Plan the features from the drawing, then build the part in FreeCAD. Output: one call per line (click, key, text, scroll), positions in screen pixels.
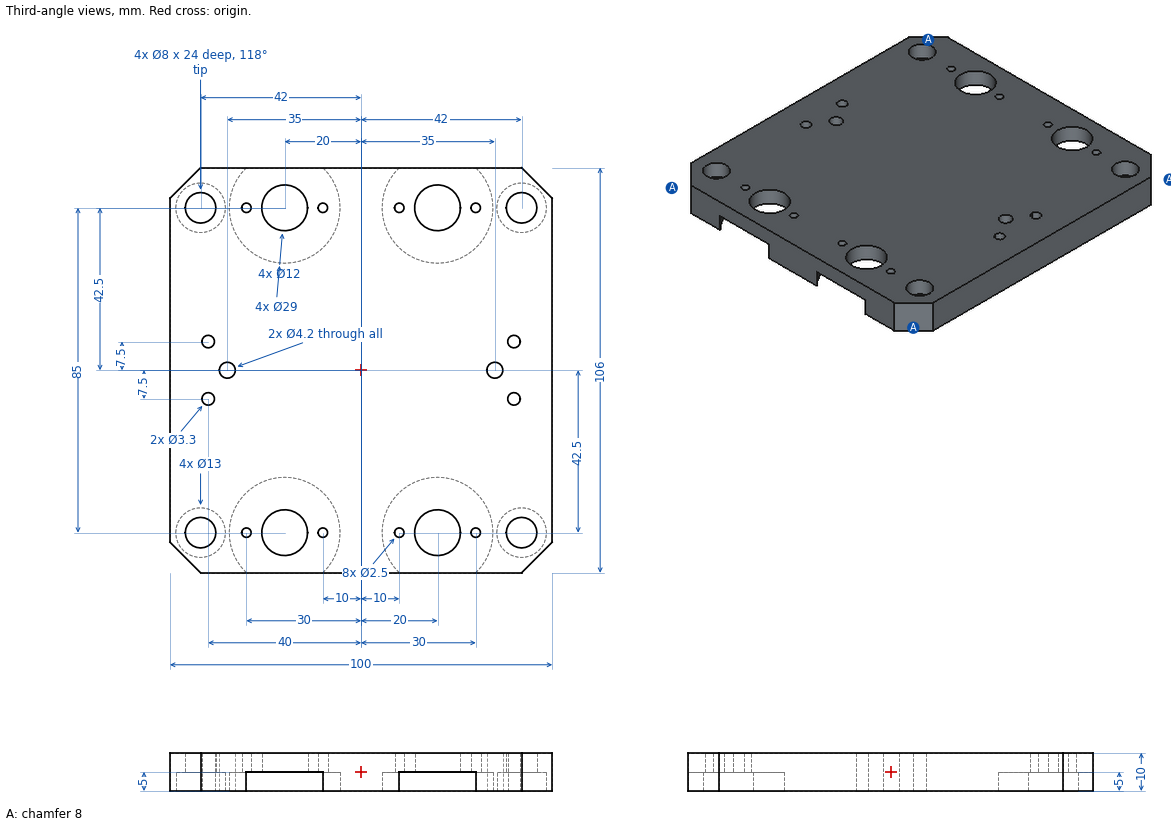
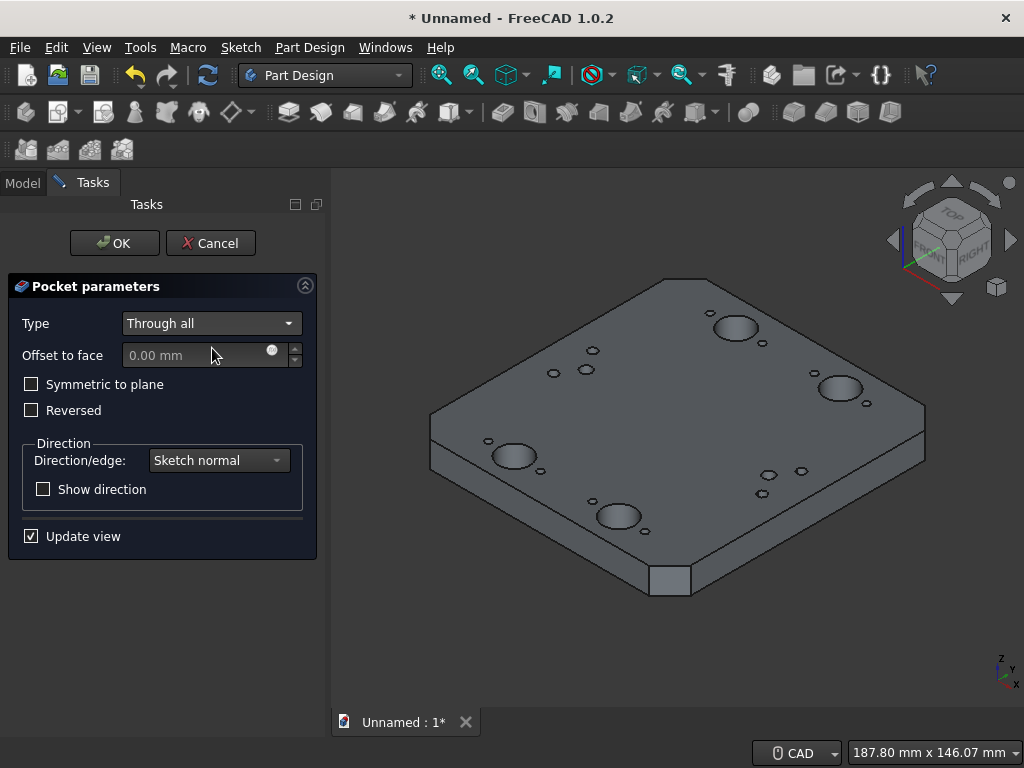
click(115, 243)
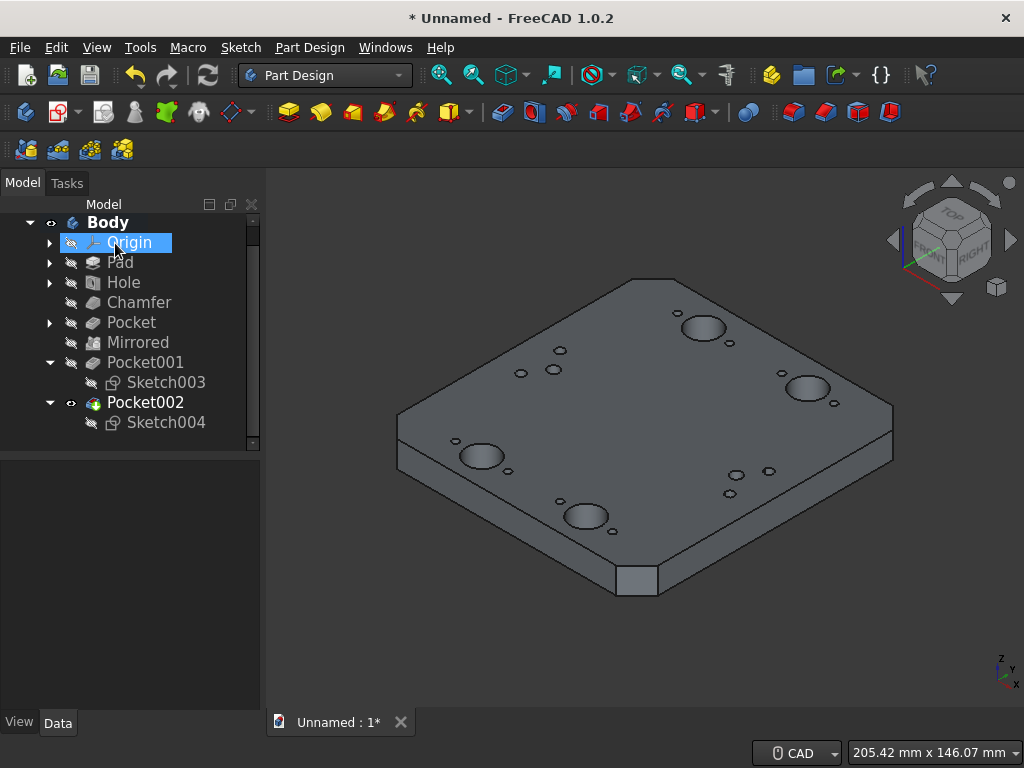
key(5)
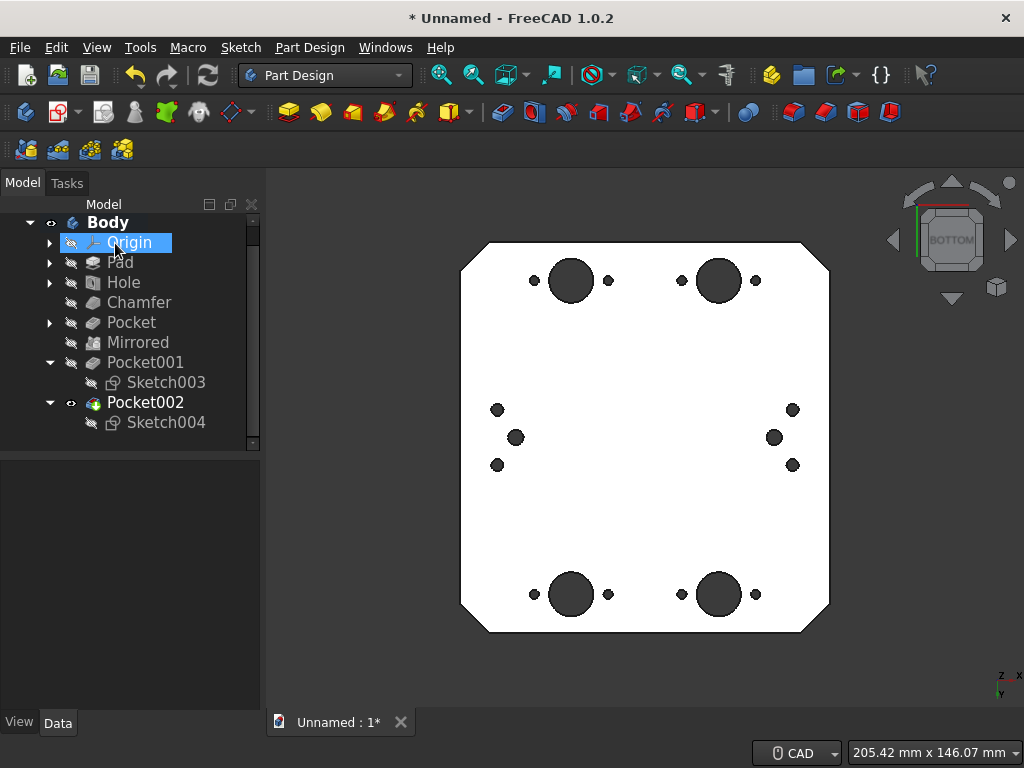
click(645, 437)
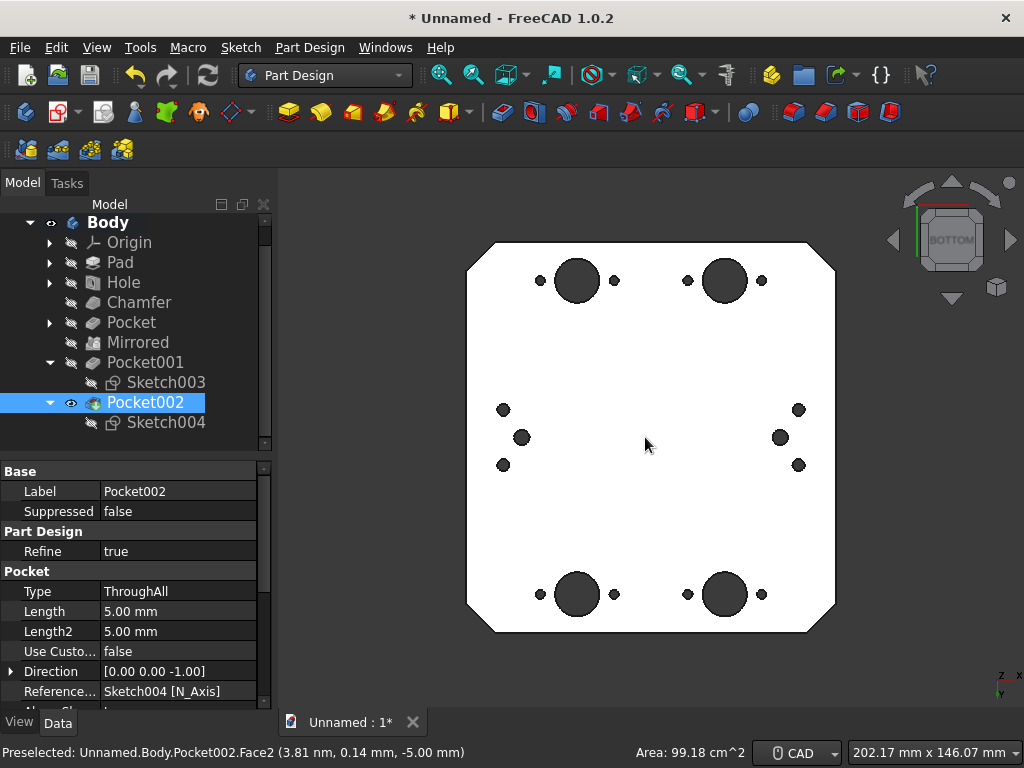
click(58, 112)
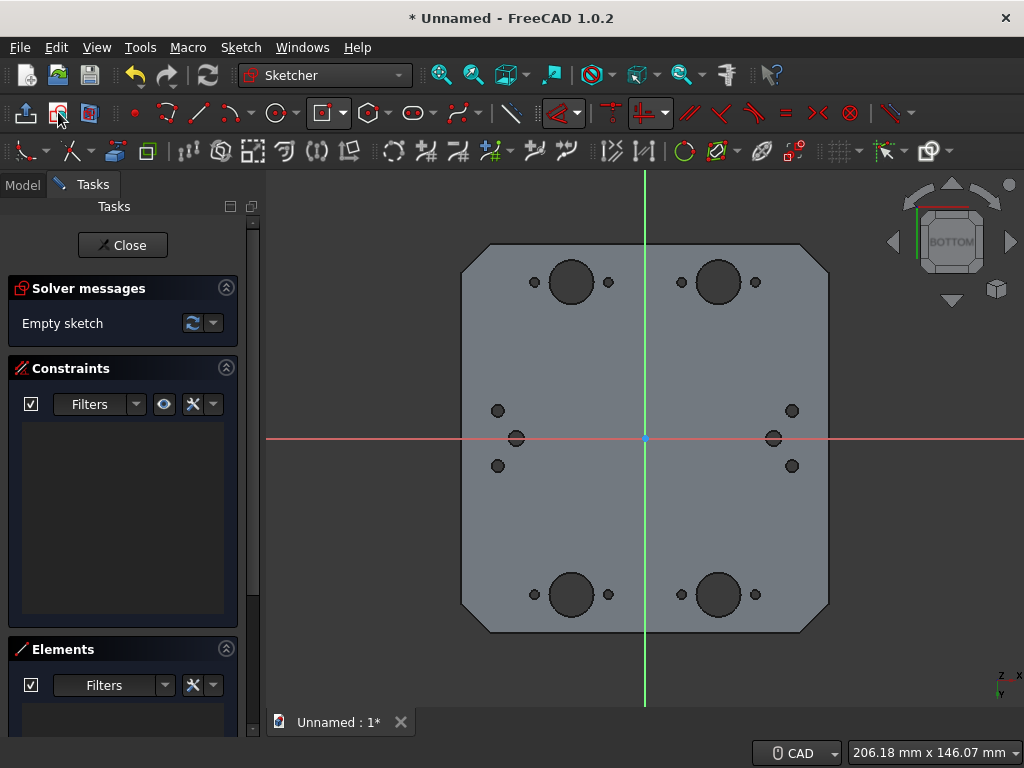
click(276, 114)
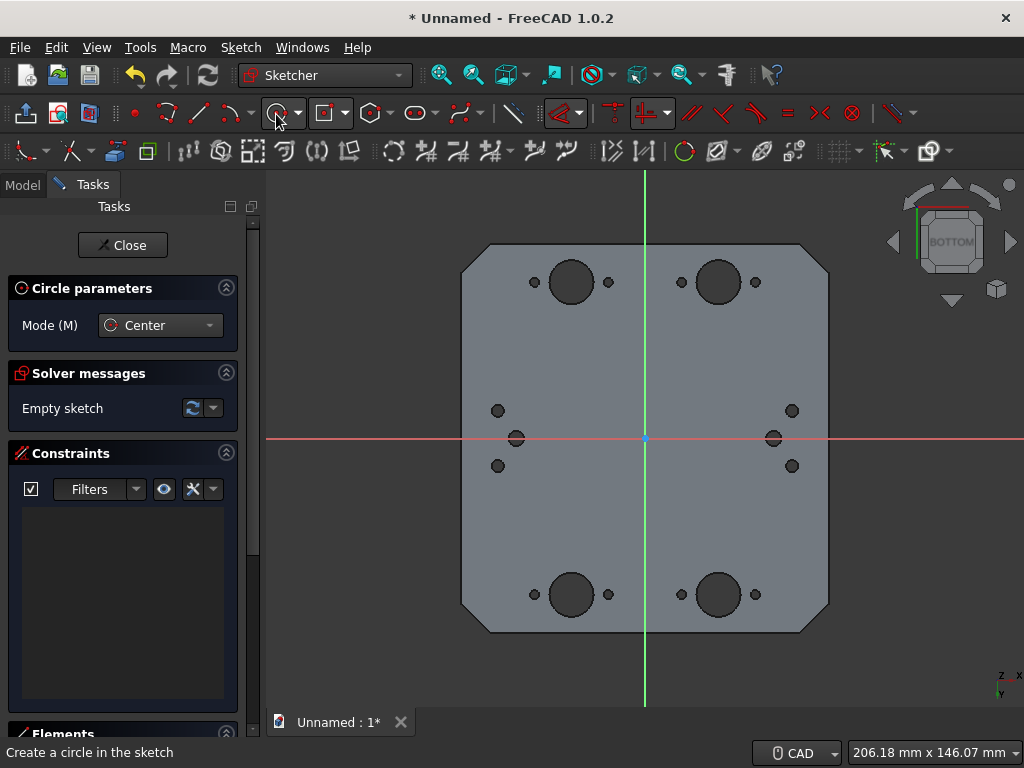
click(571, 595)
move(609, 557)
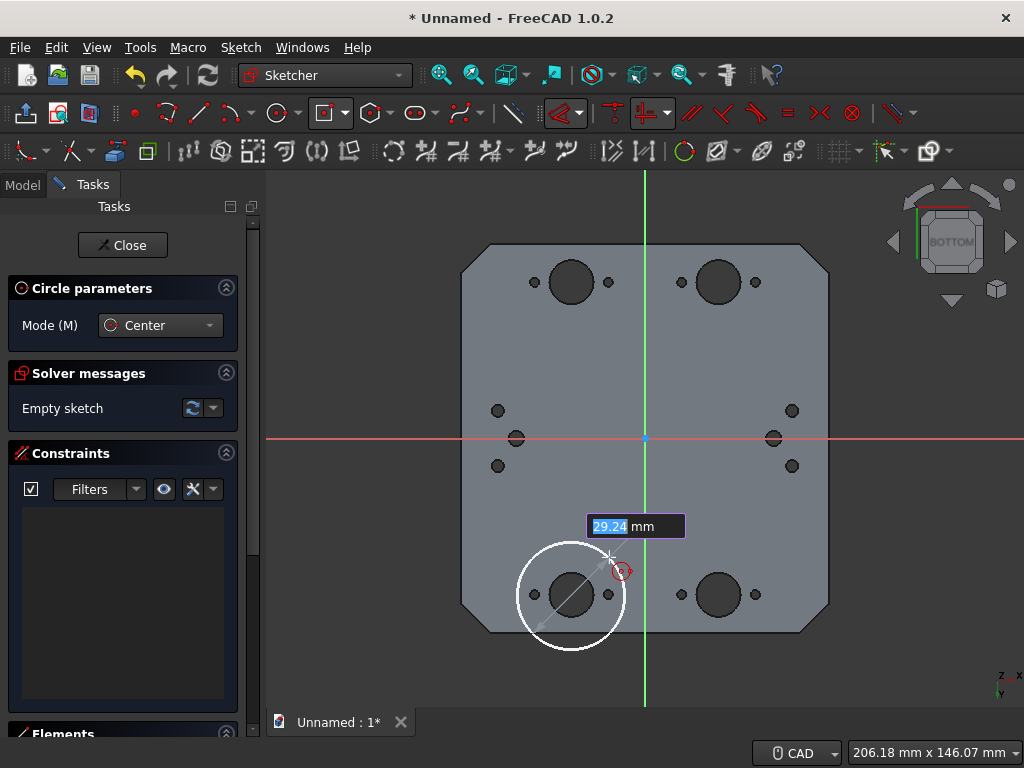
text(29)
key(Return)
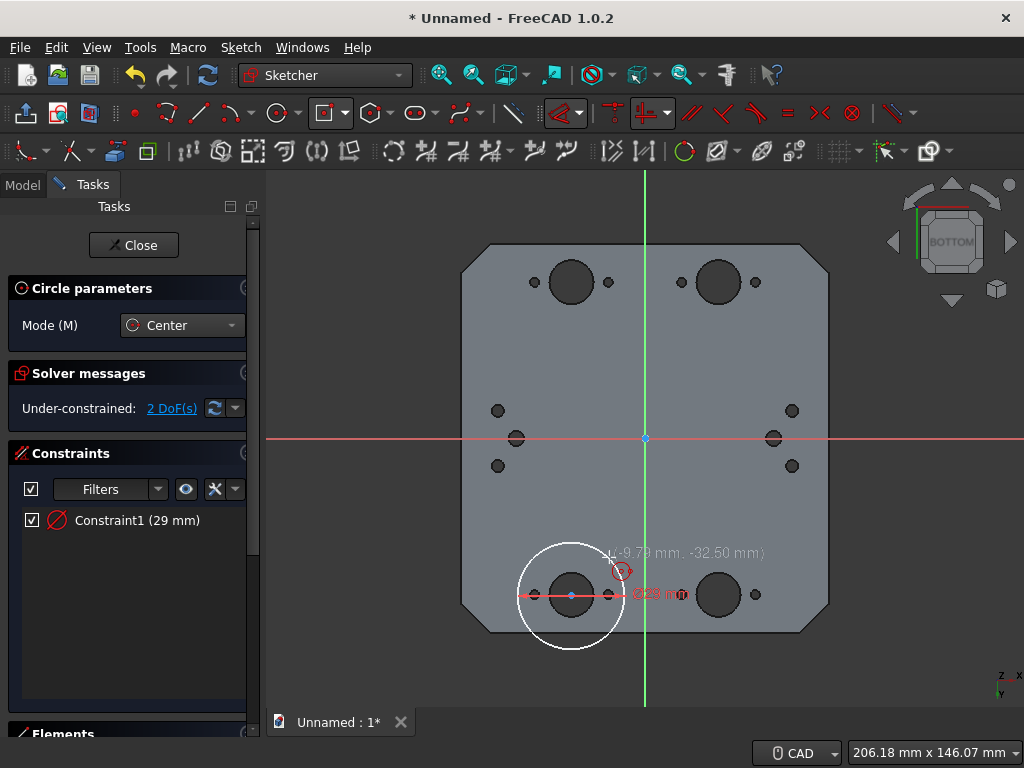
click(571, 282)
move(609, 245)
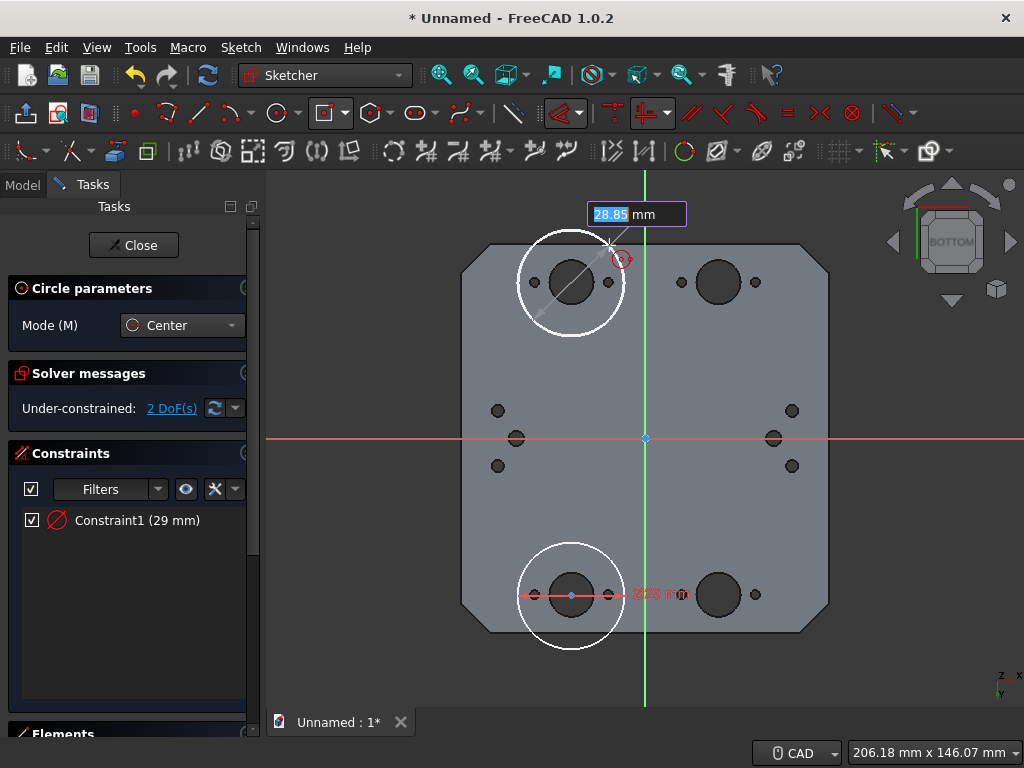
text(29)
key(Return)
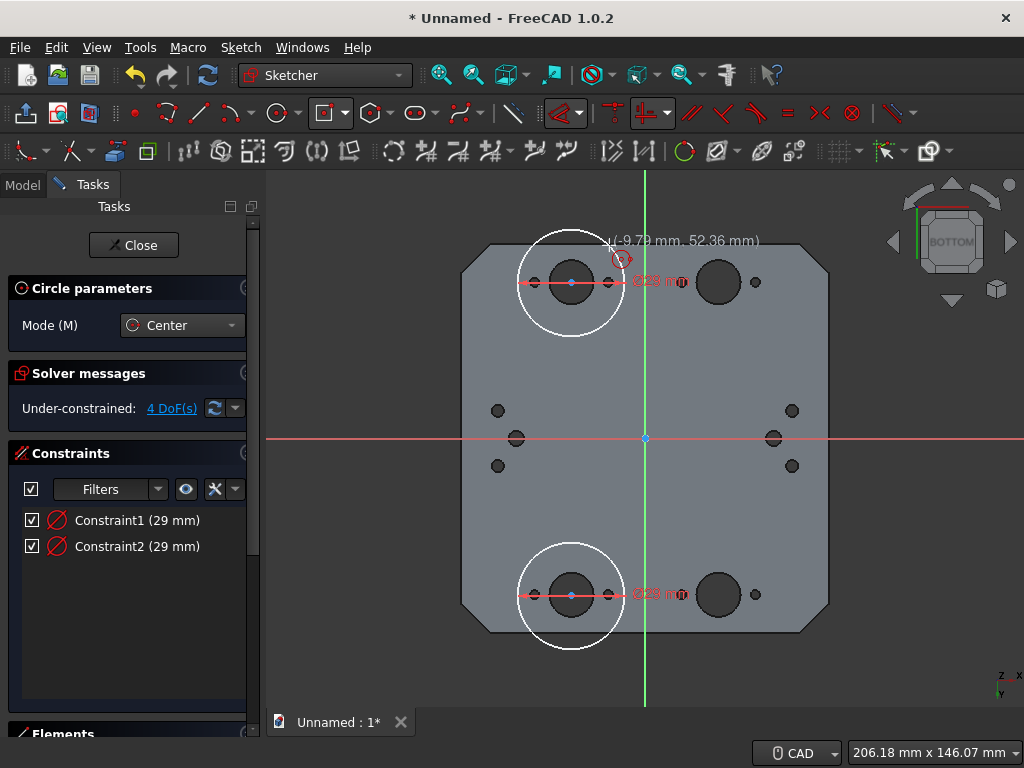
click(719, 282)
move(756, 245)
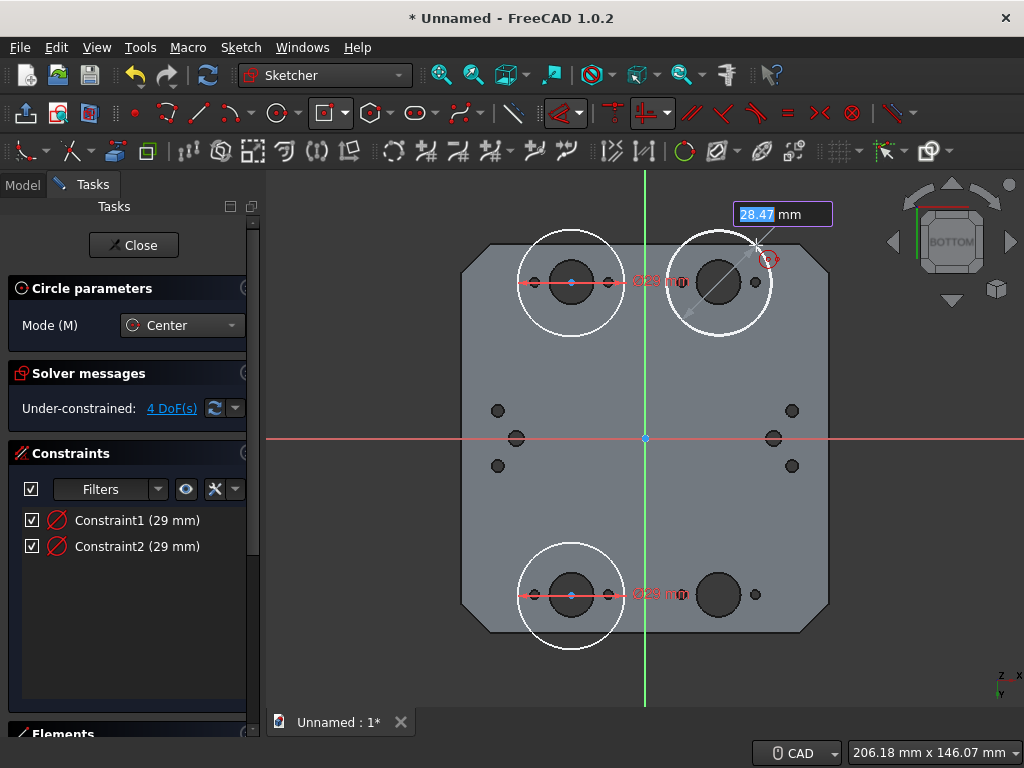
text(29)
key(Return)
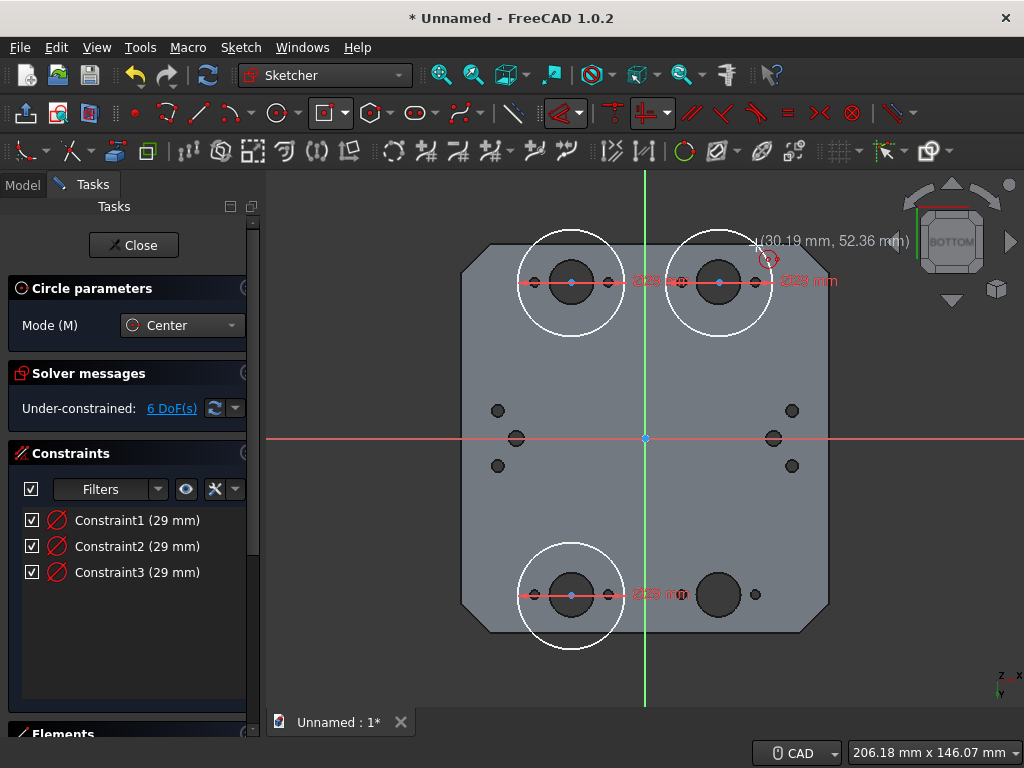
click(719, 595)
move(756, 557)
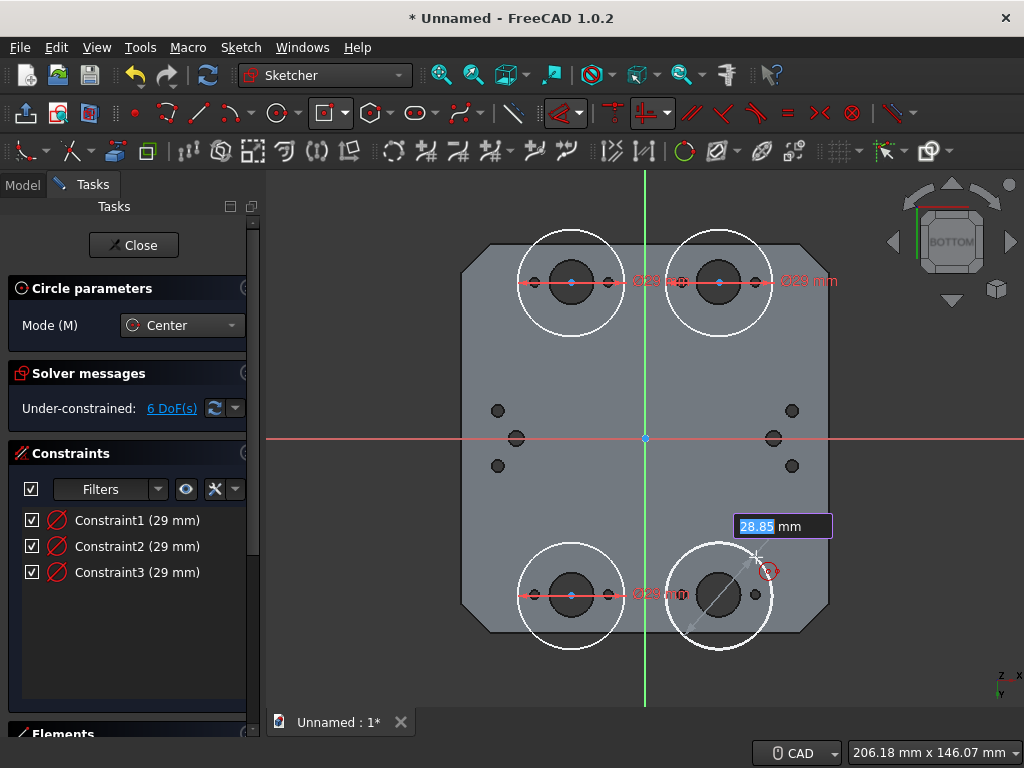
text(29)
key(Return)
key(Escape)